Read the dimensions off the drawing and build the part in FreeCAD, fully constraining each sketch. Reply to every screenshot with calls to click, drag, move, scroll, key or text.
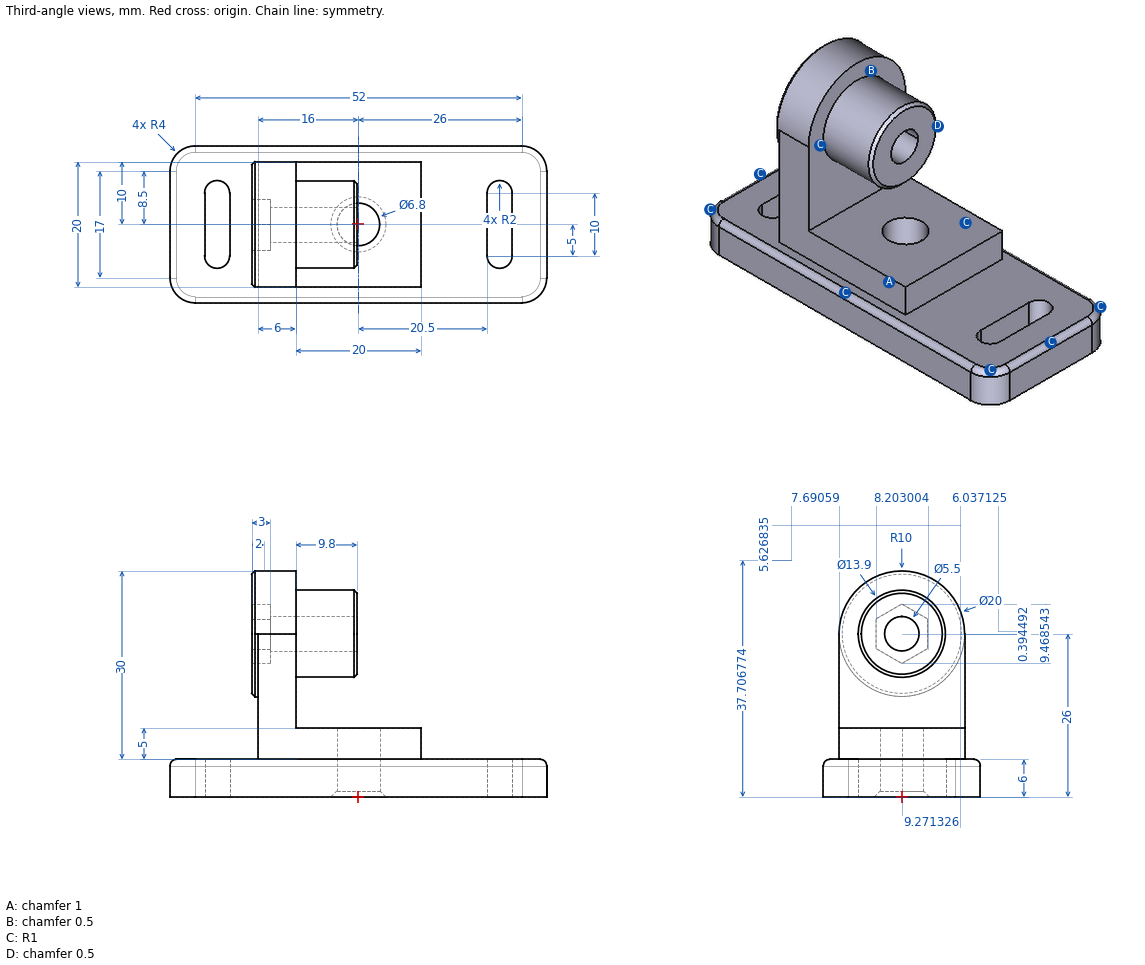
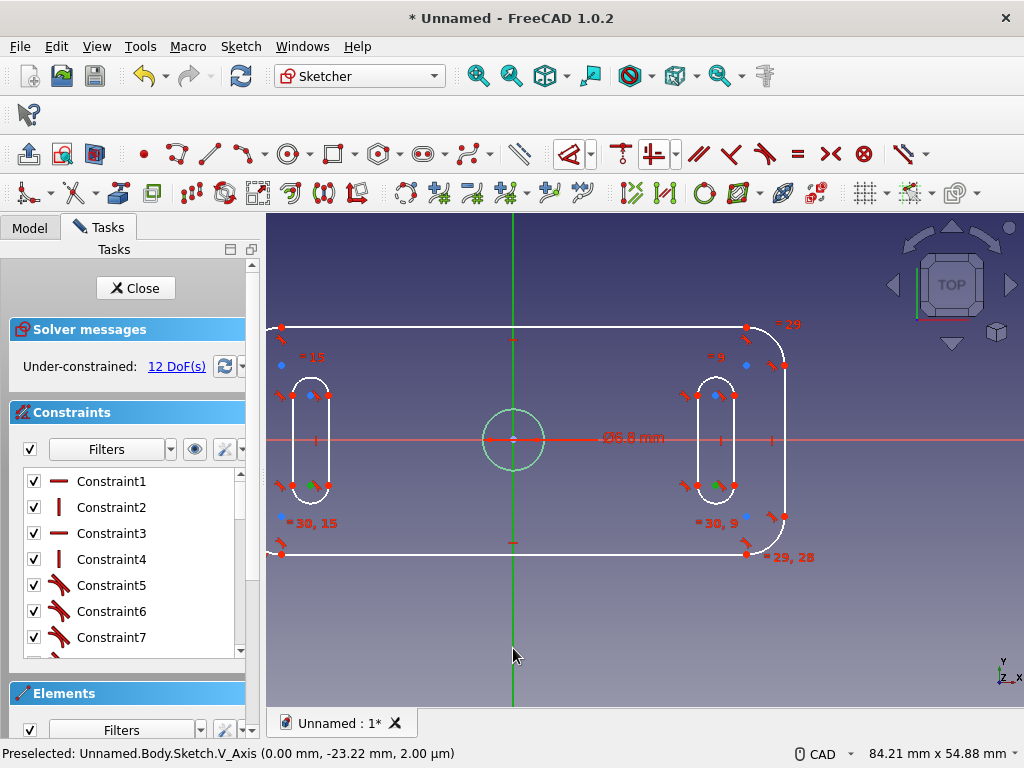
click(831, 154)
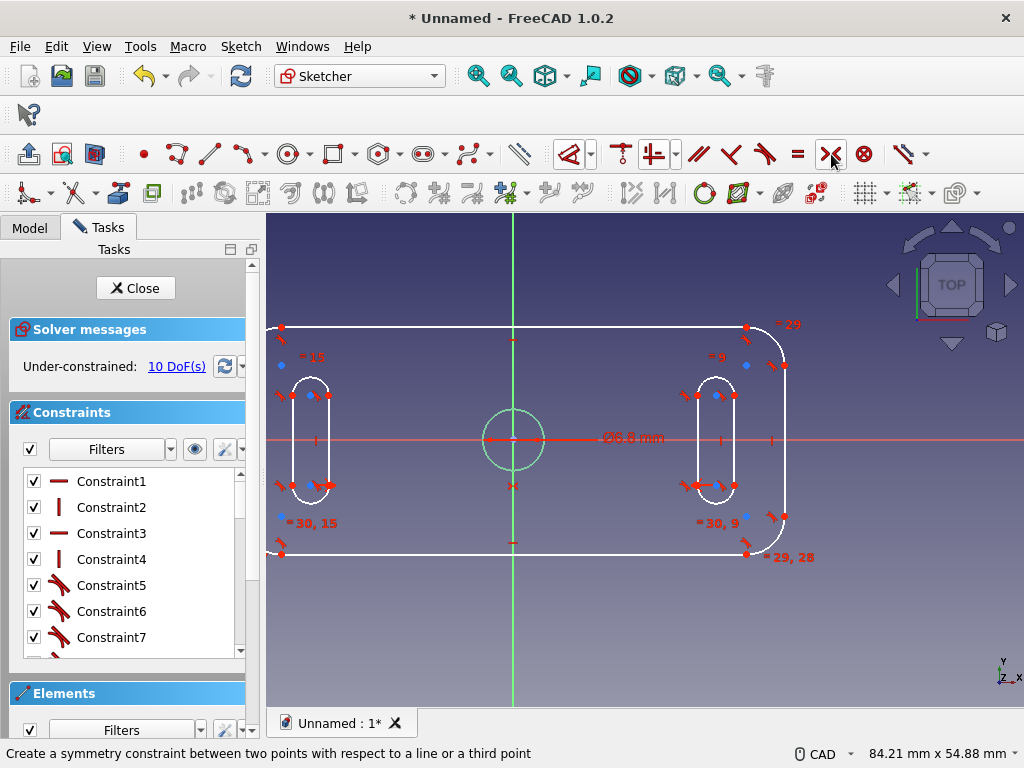
scroll(705, 501, down, 2)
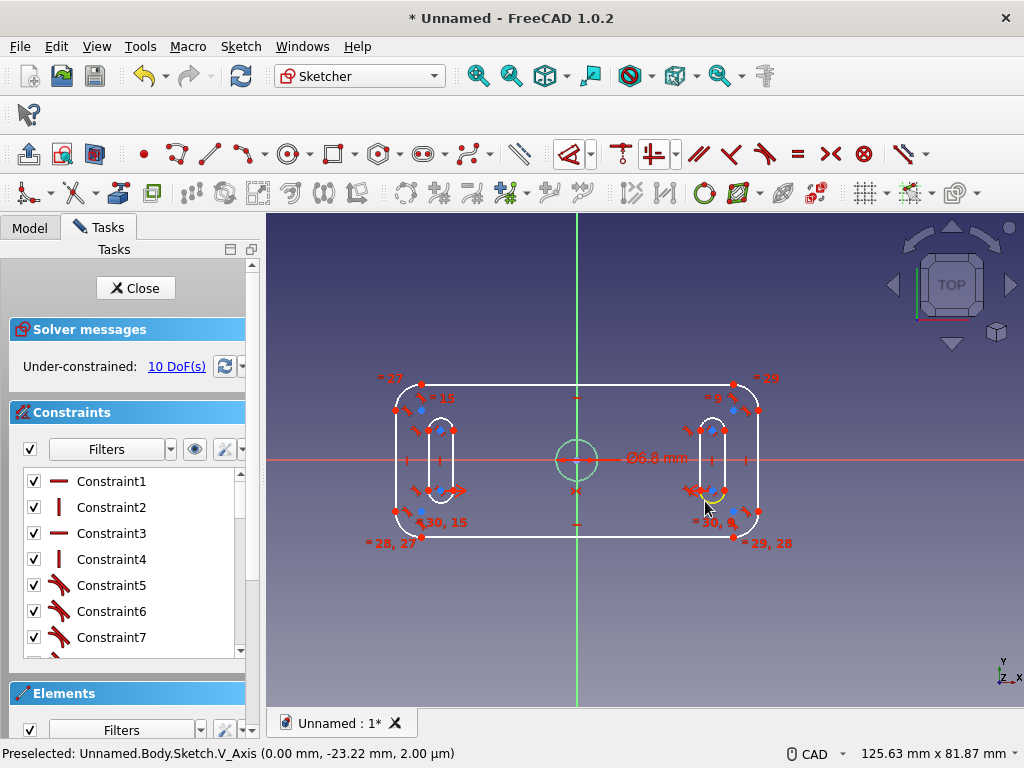
scroll(410, 388, up, 3)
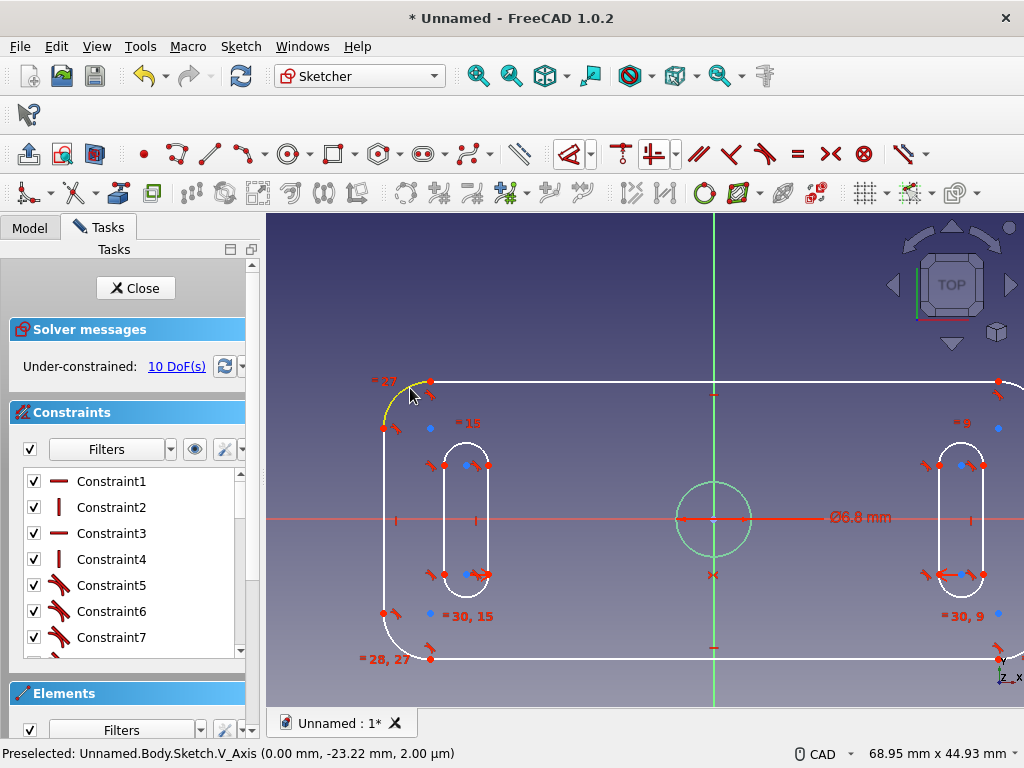
click(409, 387)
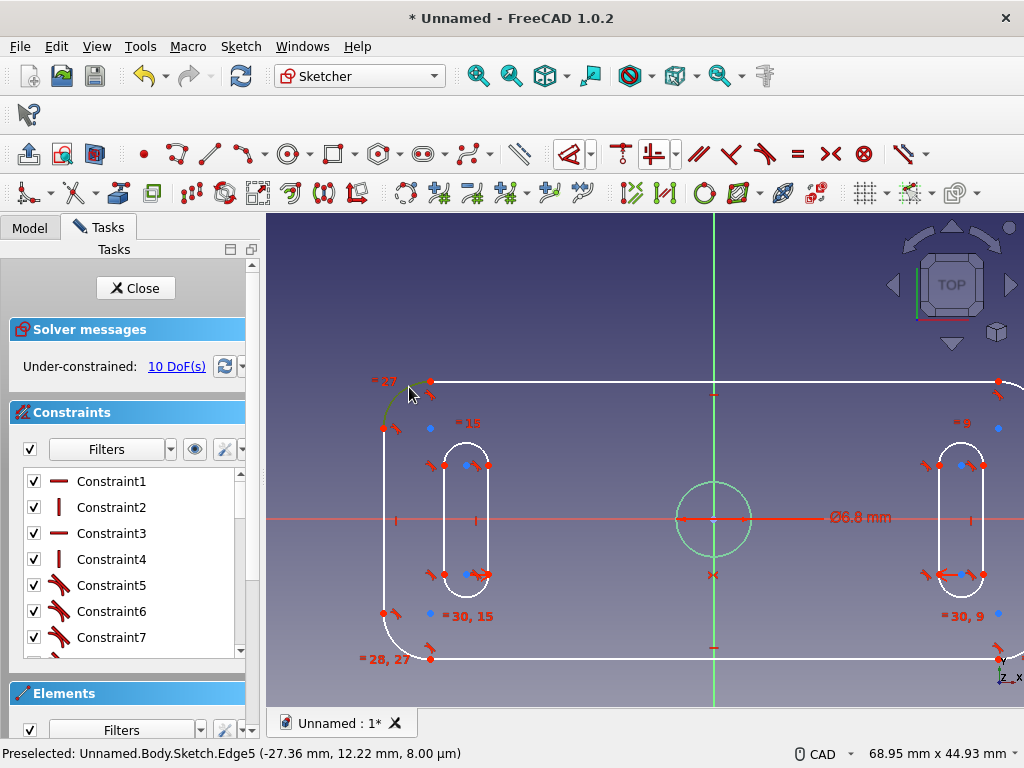
key(k)
key(r)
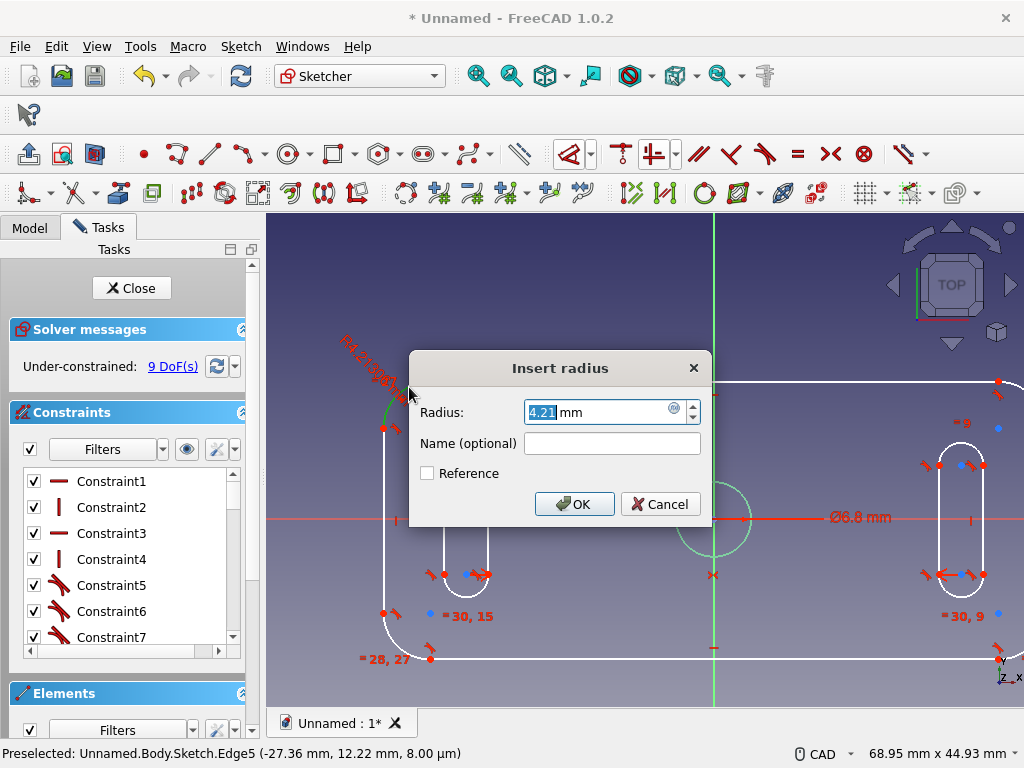
text(4)
key(Return)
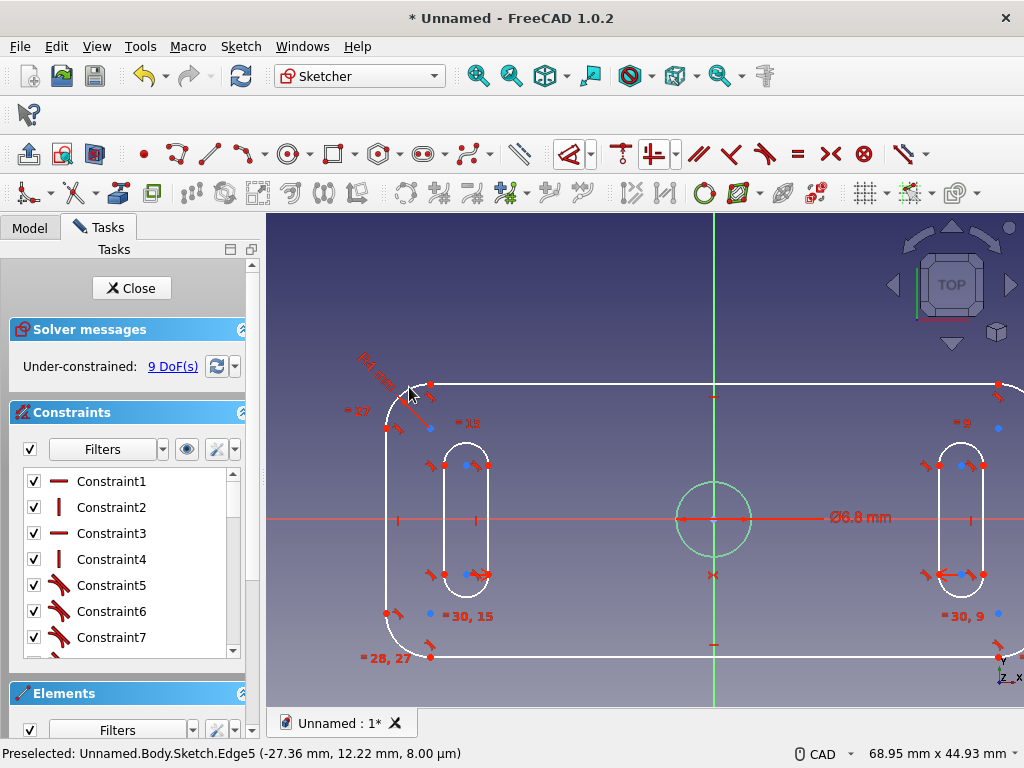
scroll(410, 388, down, 3)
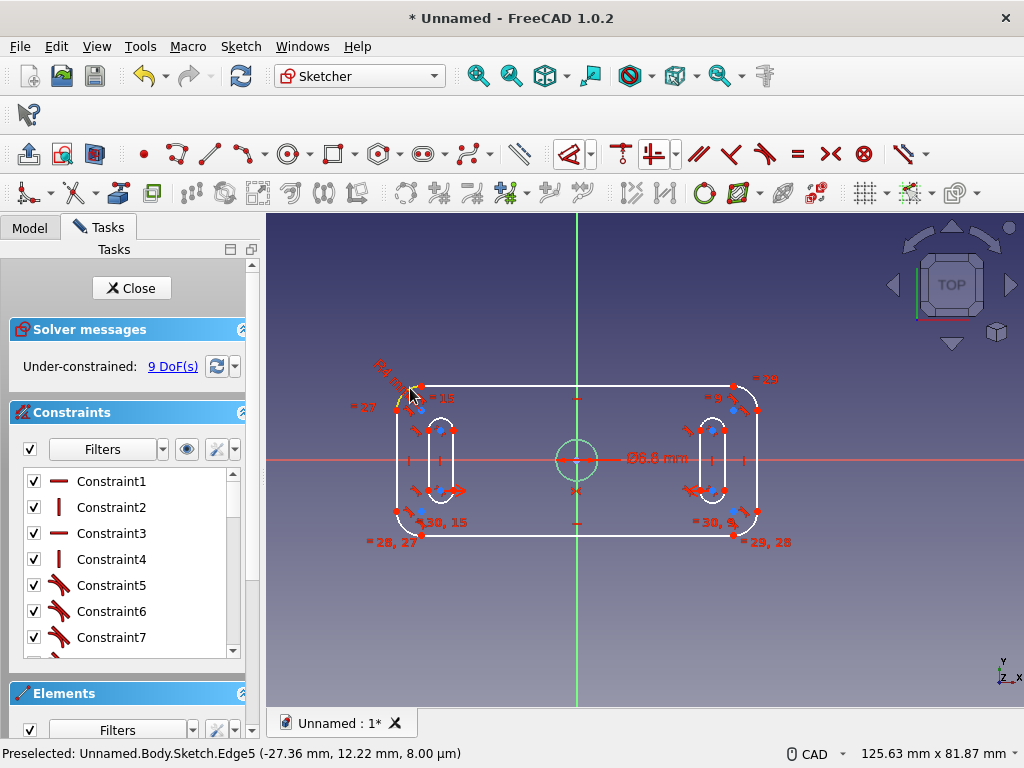
scroll(705, 501, up, 6)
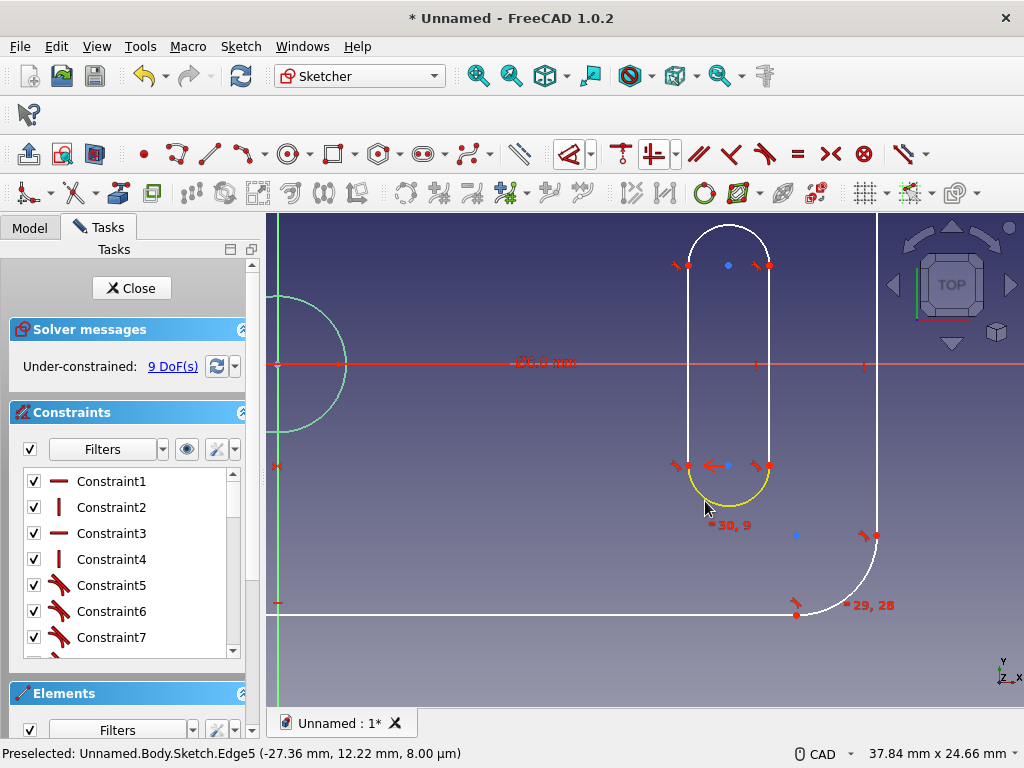
click(705, 498)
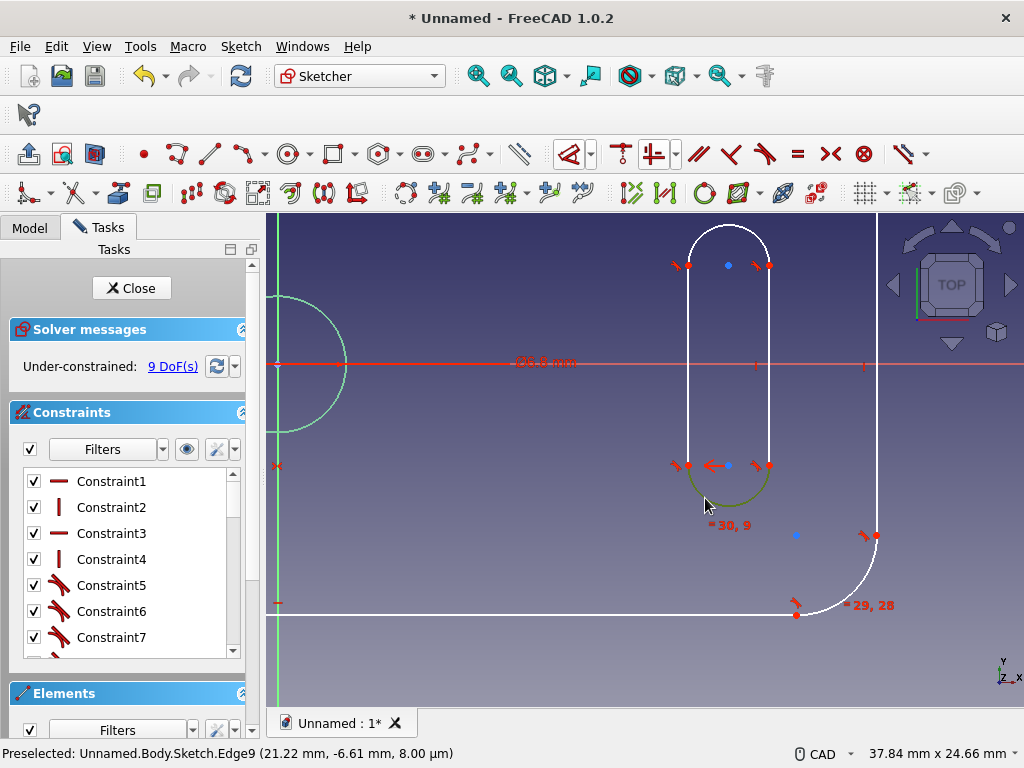
click(590, 154)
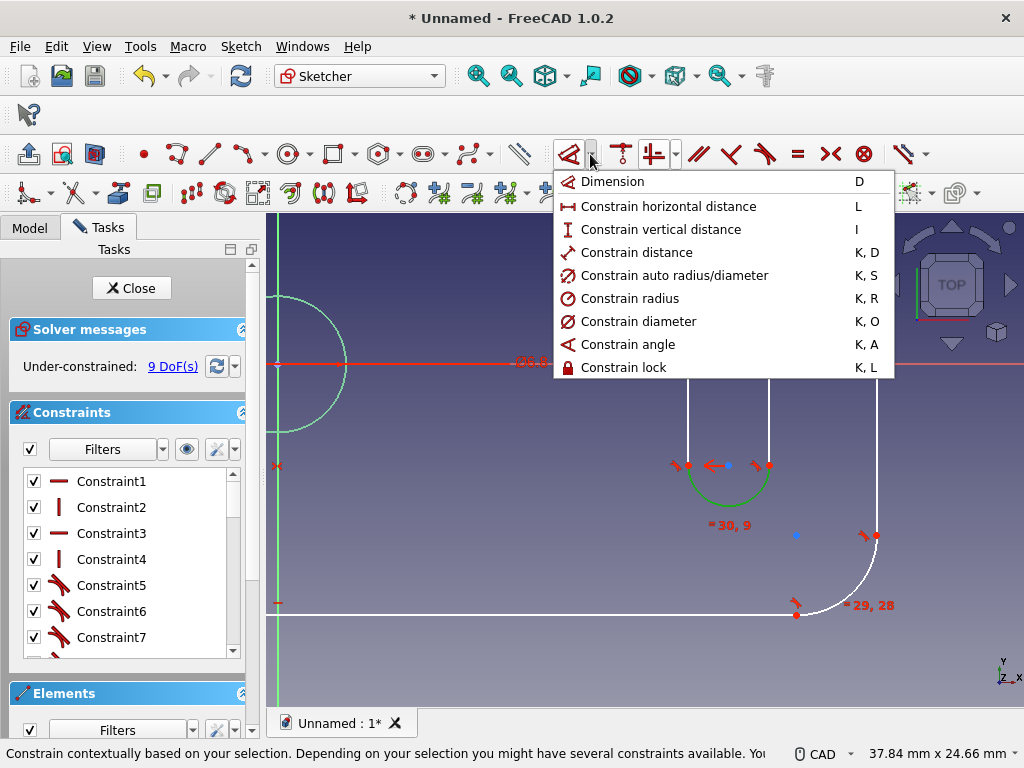
click(724, 298)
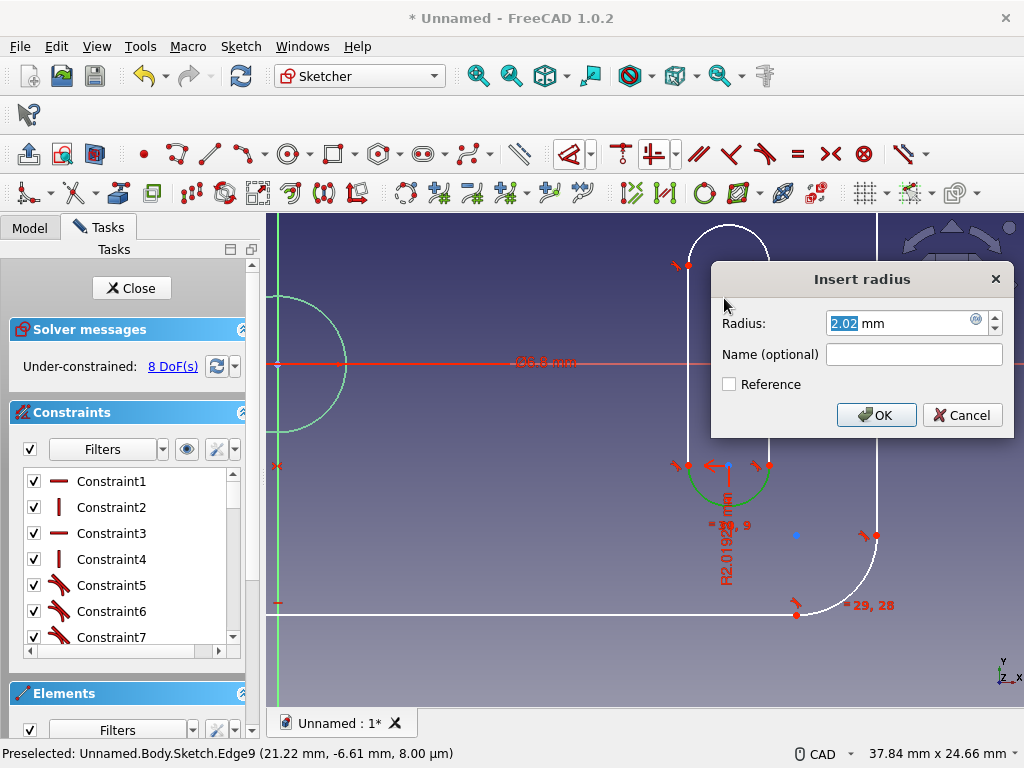
text(2)
key(Return)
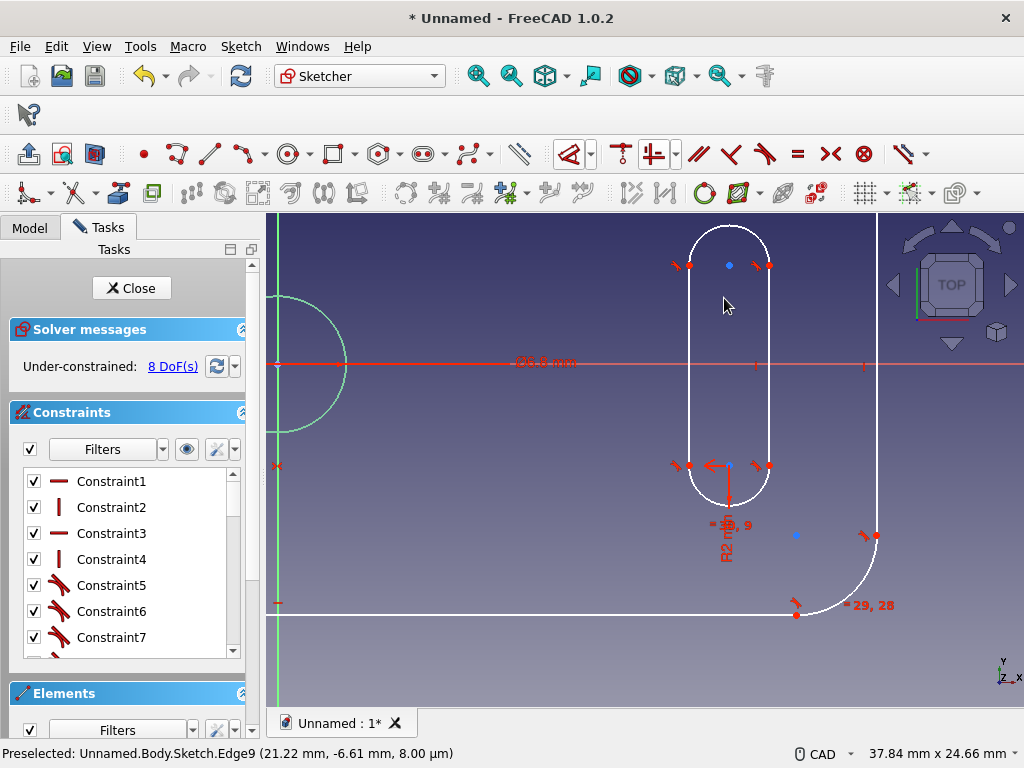
scroll(705, 501, down, 6)